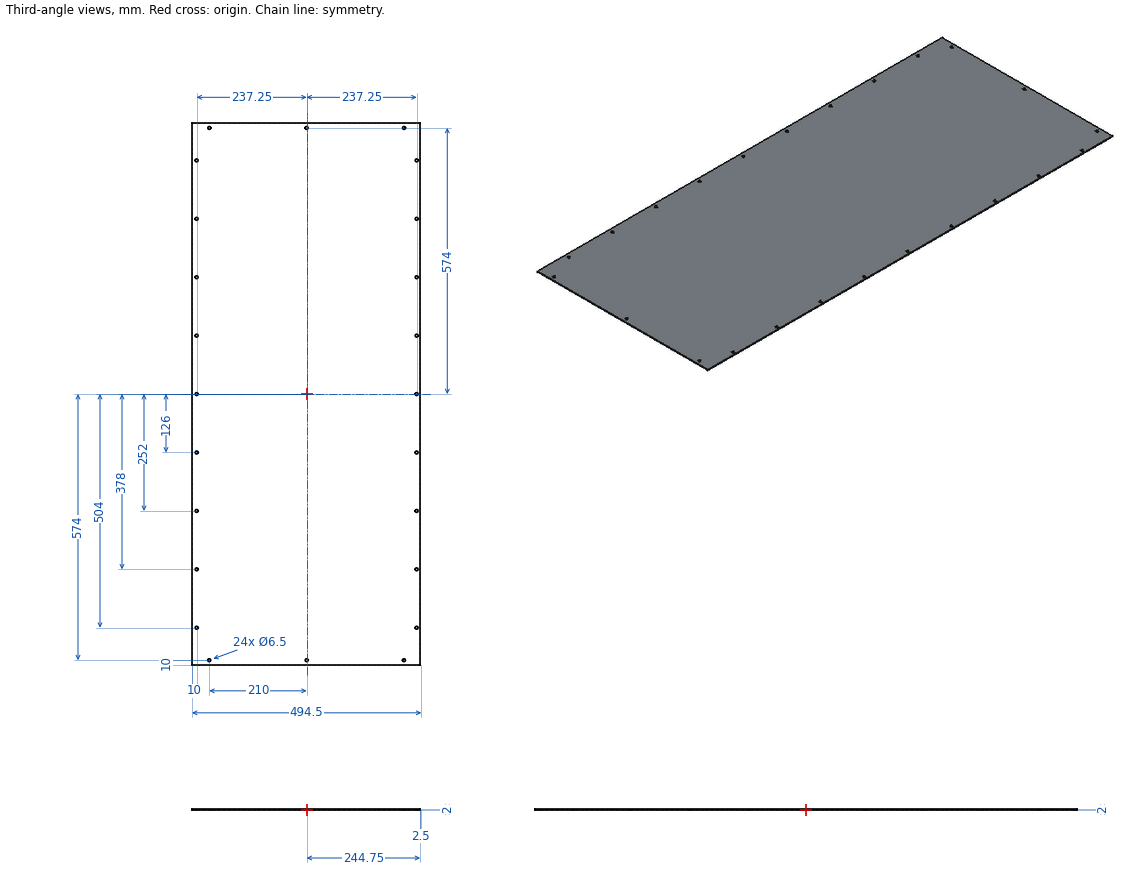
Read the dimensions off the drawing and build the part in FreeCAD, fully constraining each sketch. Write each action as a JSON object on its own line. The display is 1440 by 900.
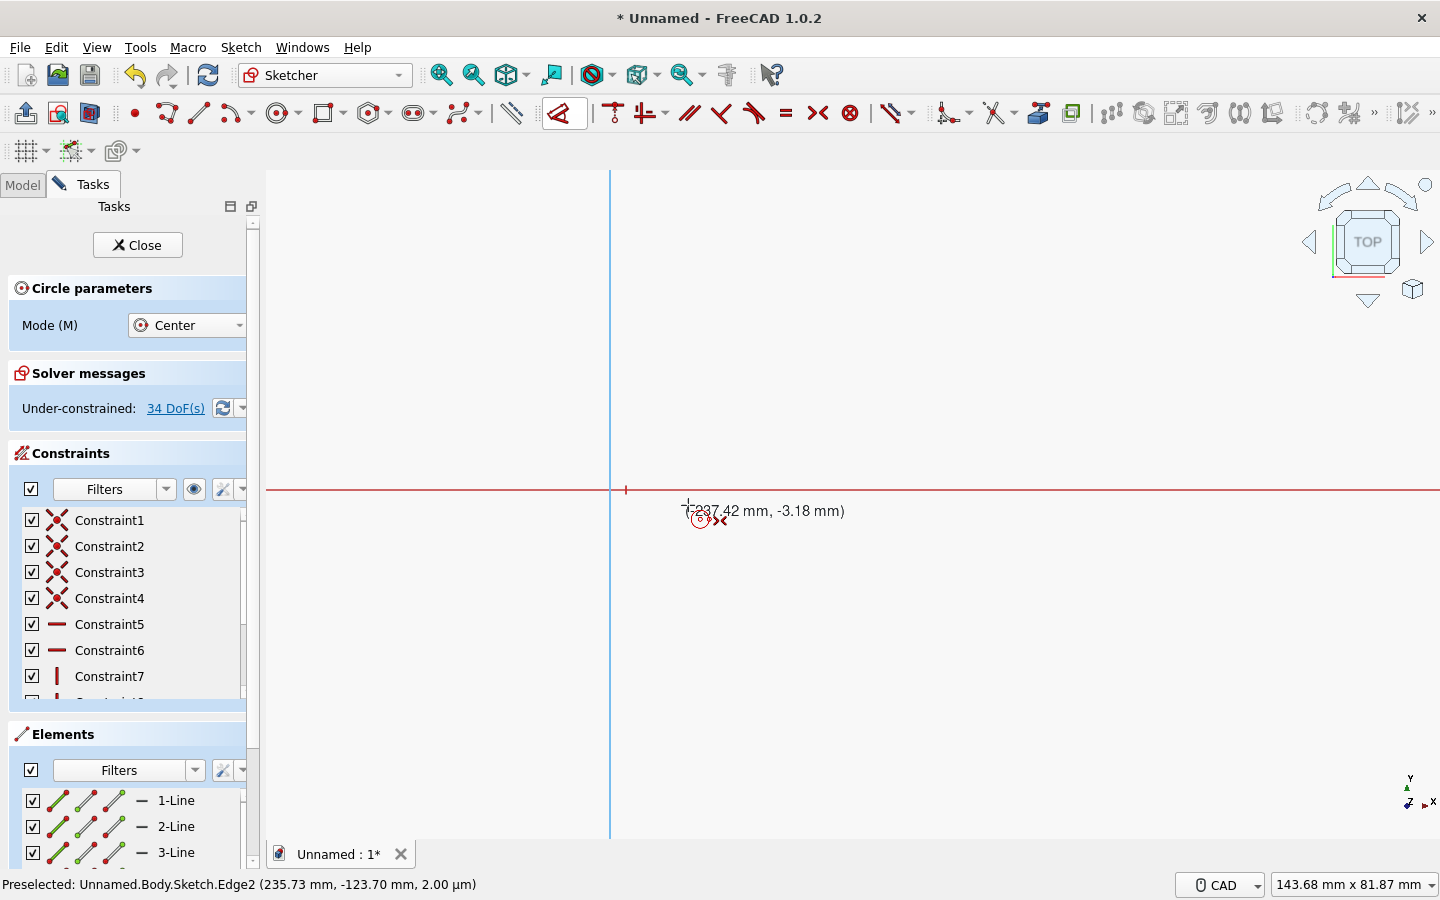
{"action": "scroll", "coordinate": [688, 505], "scroll_direction": "down", "scroll_amount": 15}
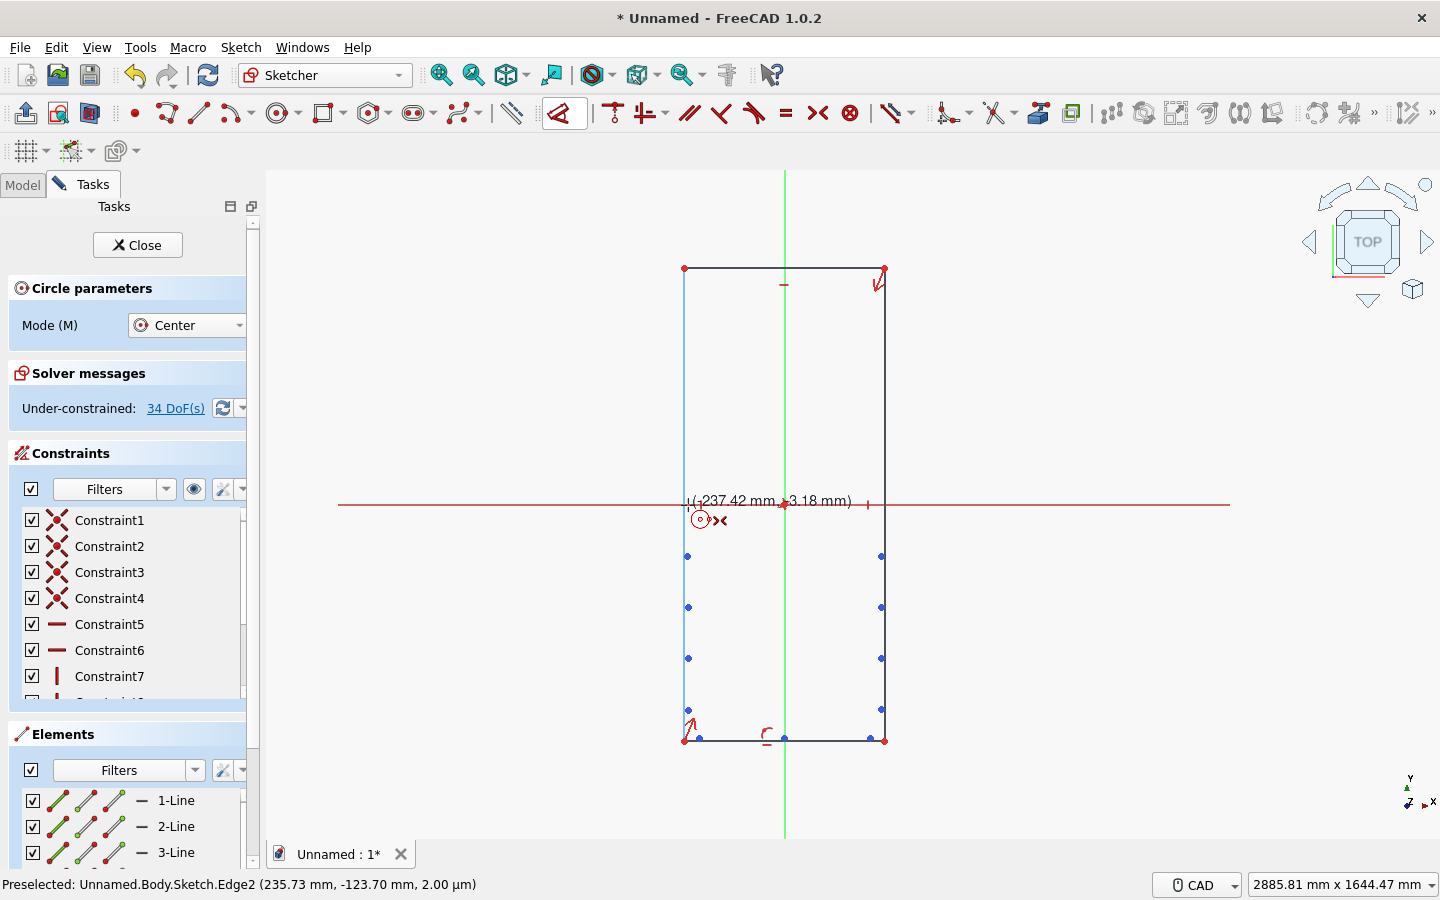
{"action": "scroll", "coordinate": [688, 505], "scroll_direction": "up", "scroll_amount": 7}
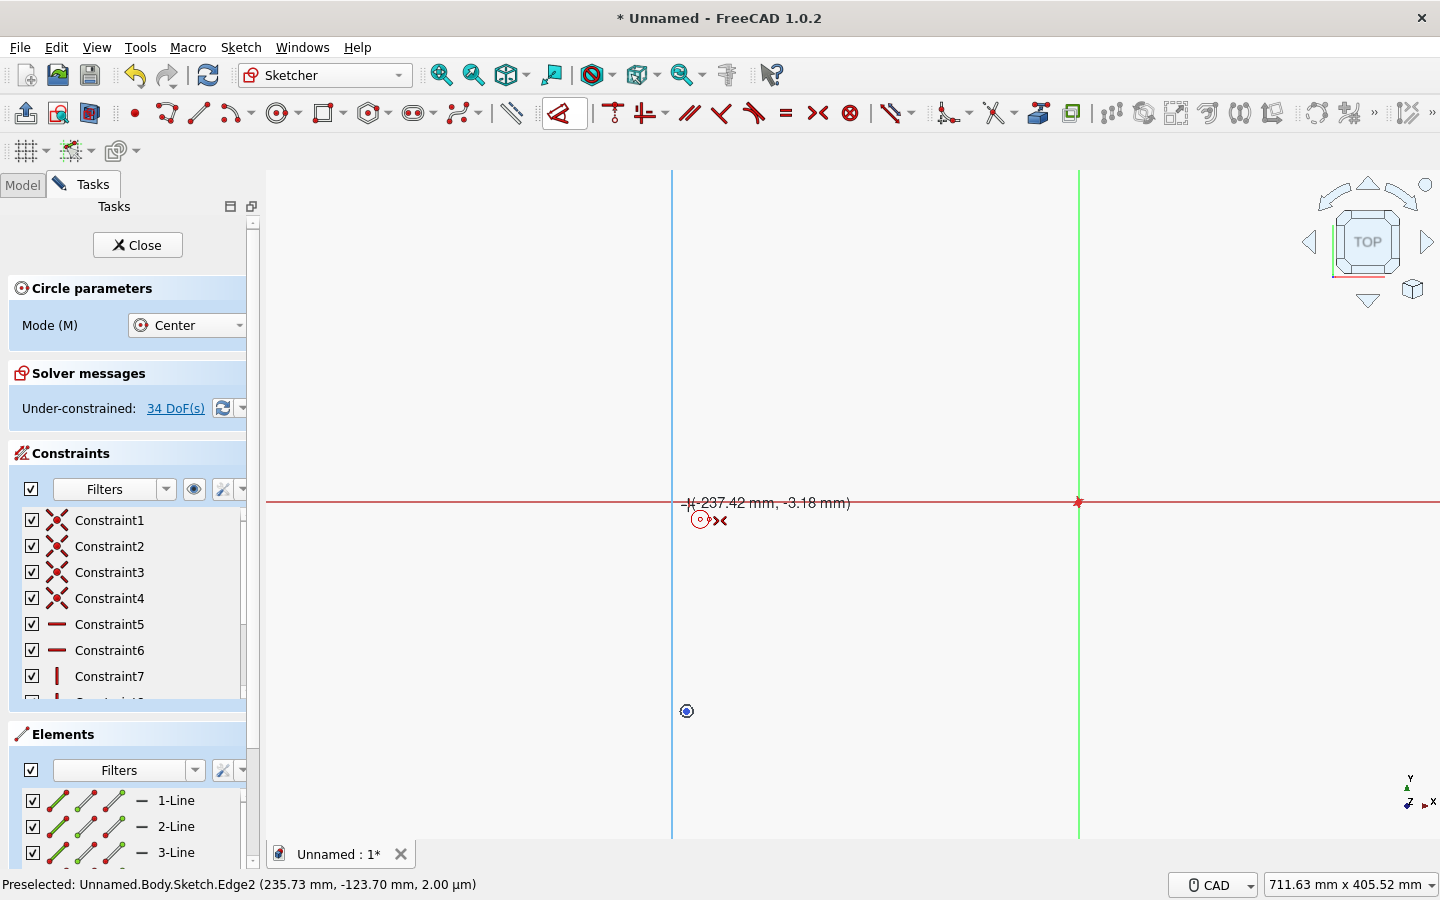
{"action": "left_click", "coordinate": [687, 502]}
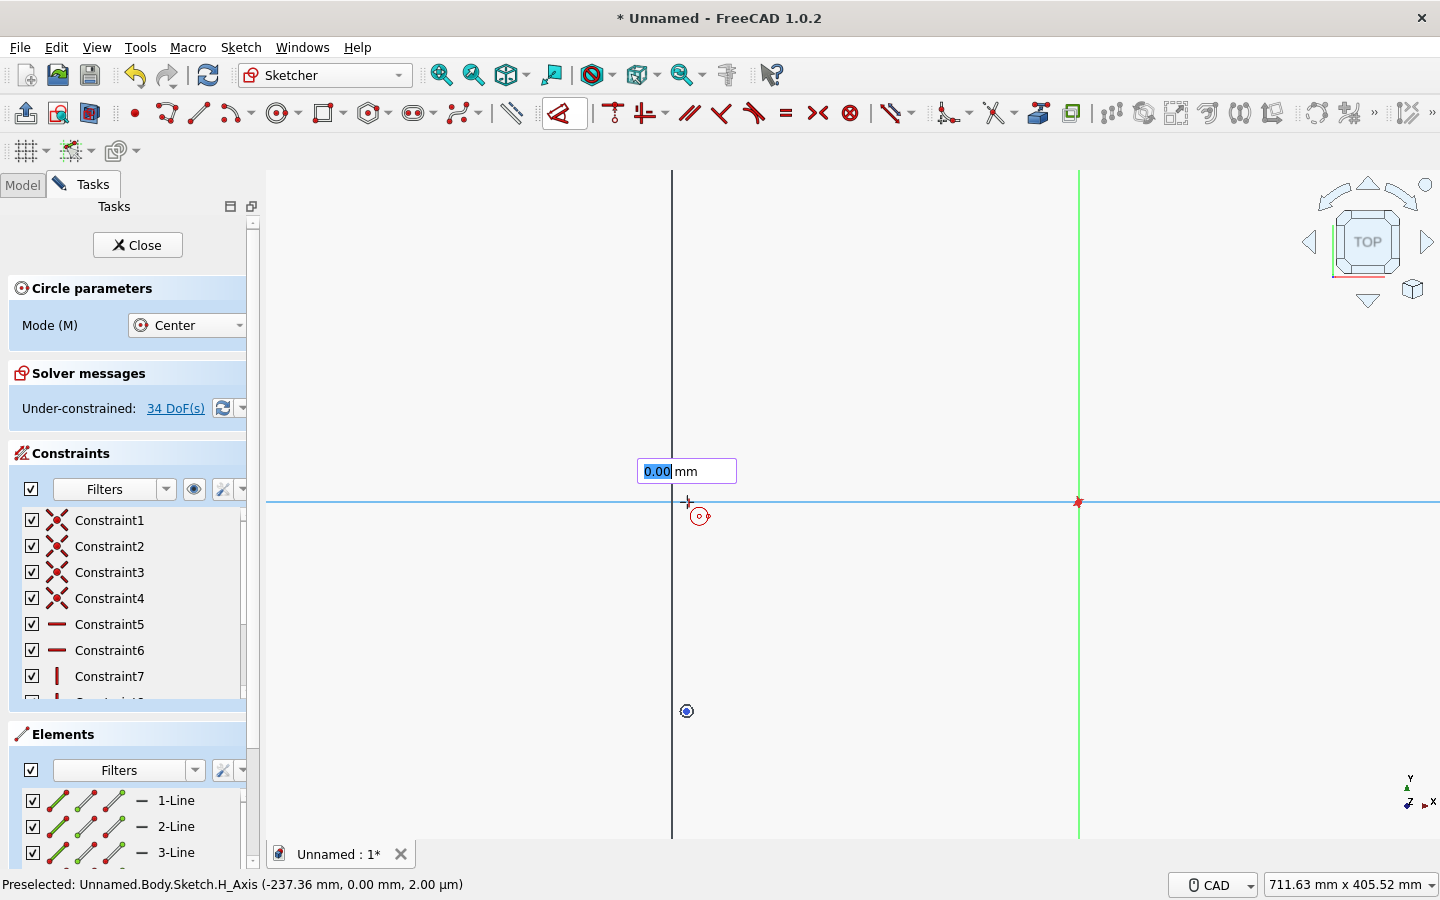
{"action": "scroll", "coordinate": [685, 507], "scroll_direction": "up", "scroll_amount": 6}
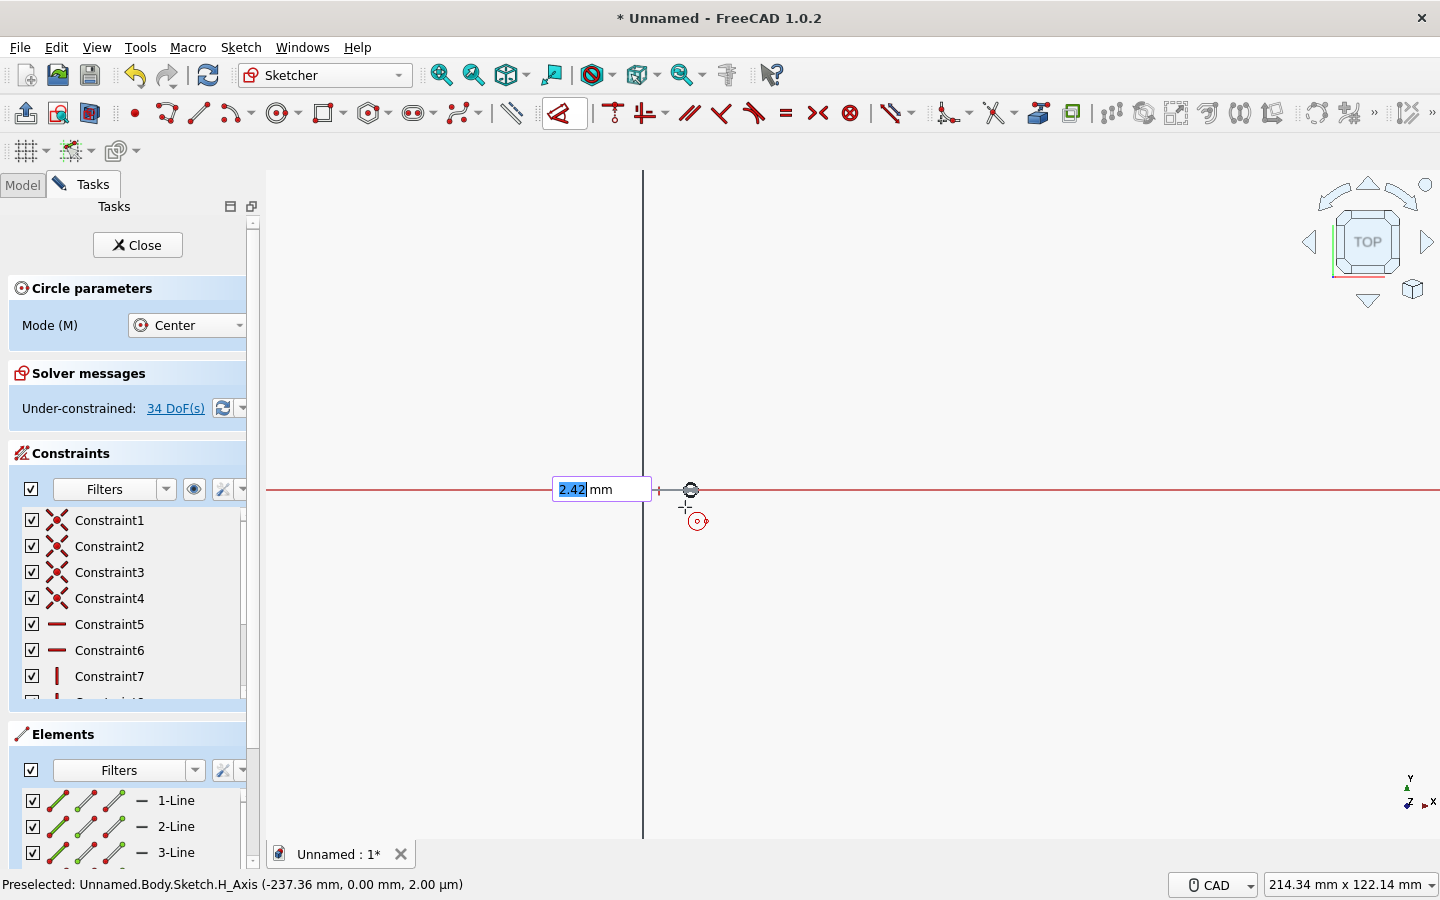
{"action": "left_click", "coordinate": [685, 507]}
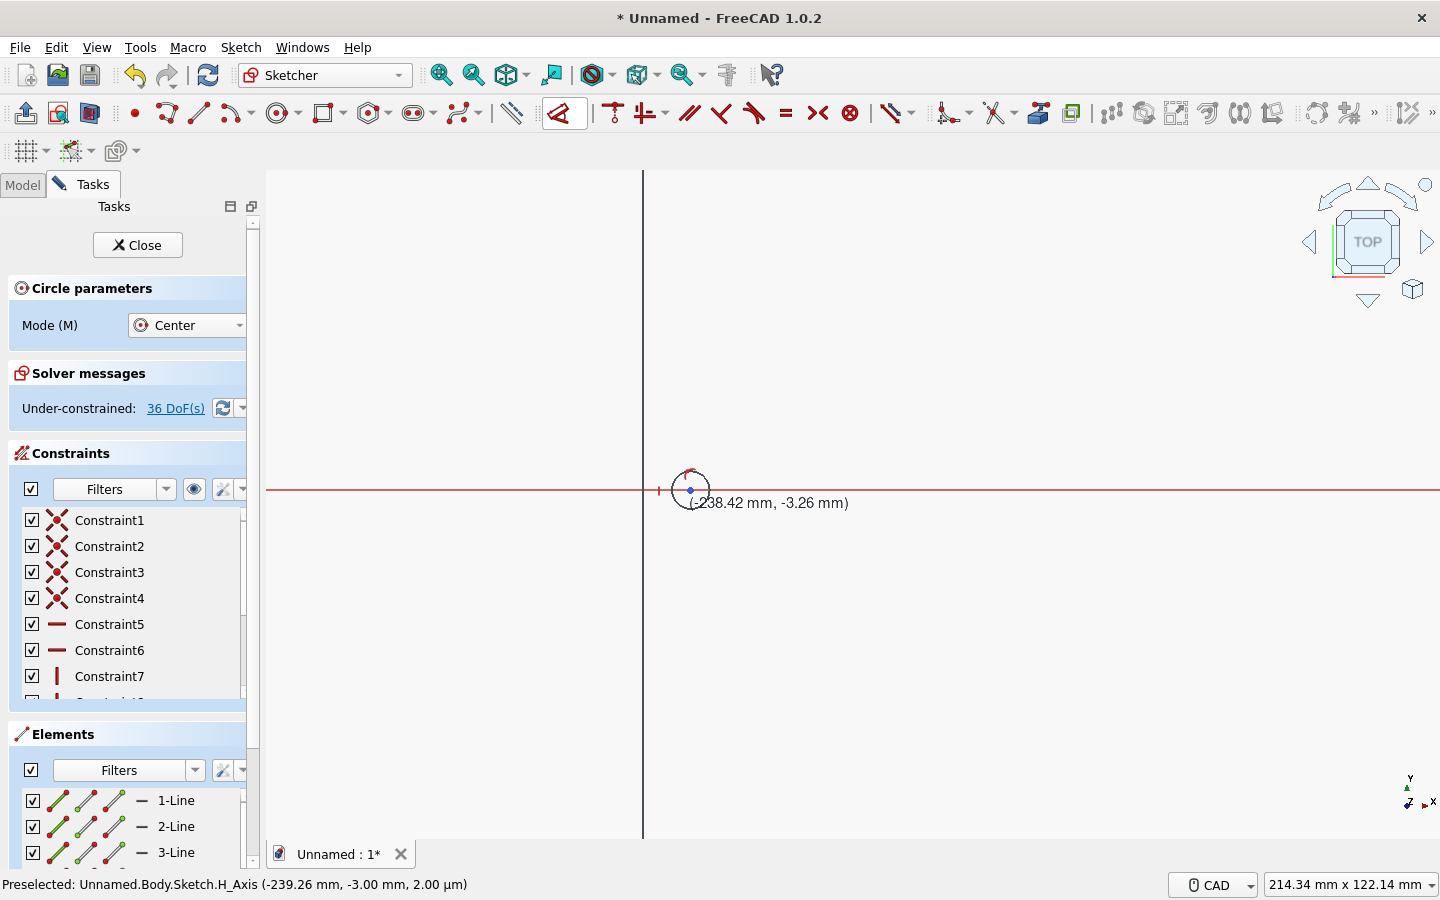
{"action": "scroll", "coordinate": [688, 506], "scroll_direction": "down", "scroll_amount": 13}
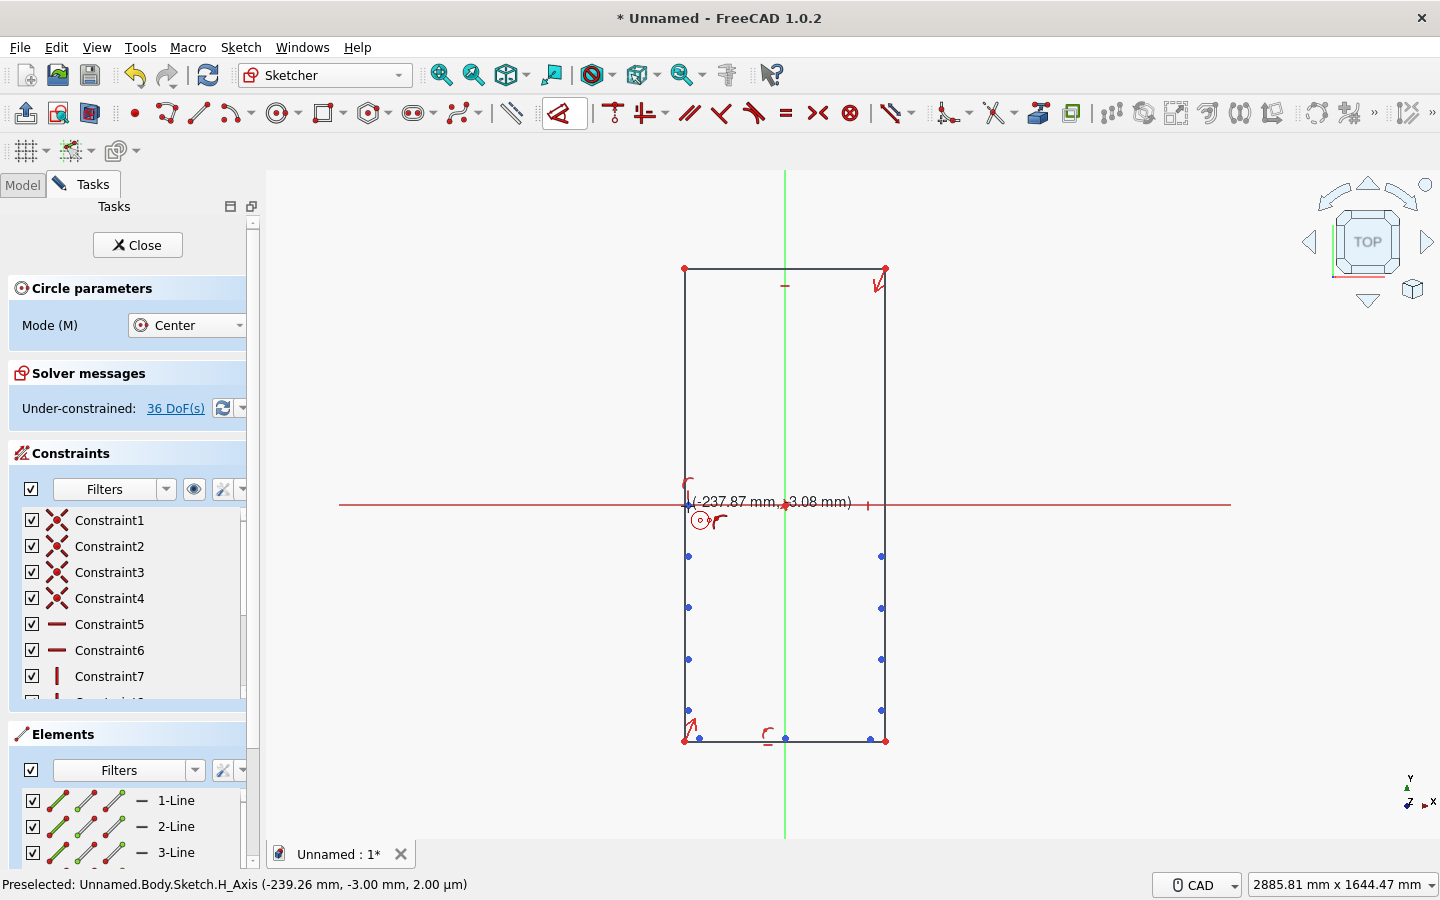
{"action": "scroll", "coordinate": [689, 454], "scroll_direction": "up", "scroll_amount": 15}